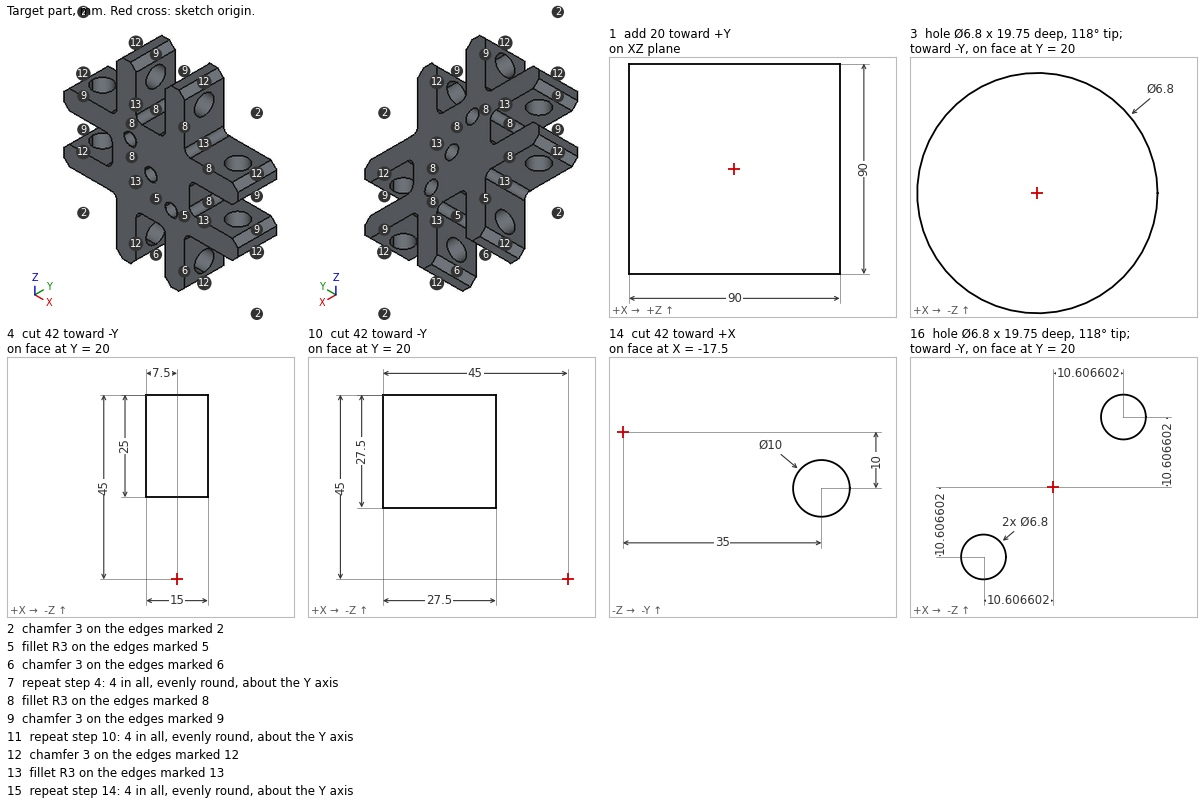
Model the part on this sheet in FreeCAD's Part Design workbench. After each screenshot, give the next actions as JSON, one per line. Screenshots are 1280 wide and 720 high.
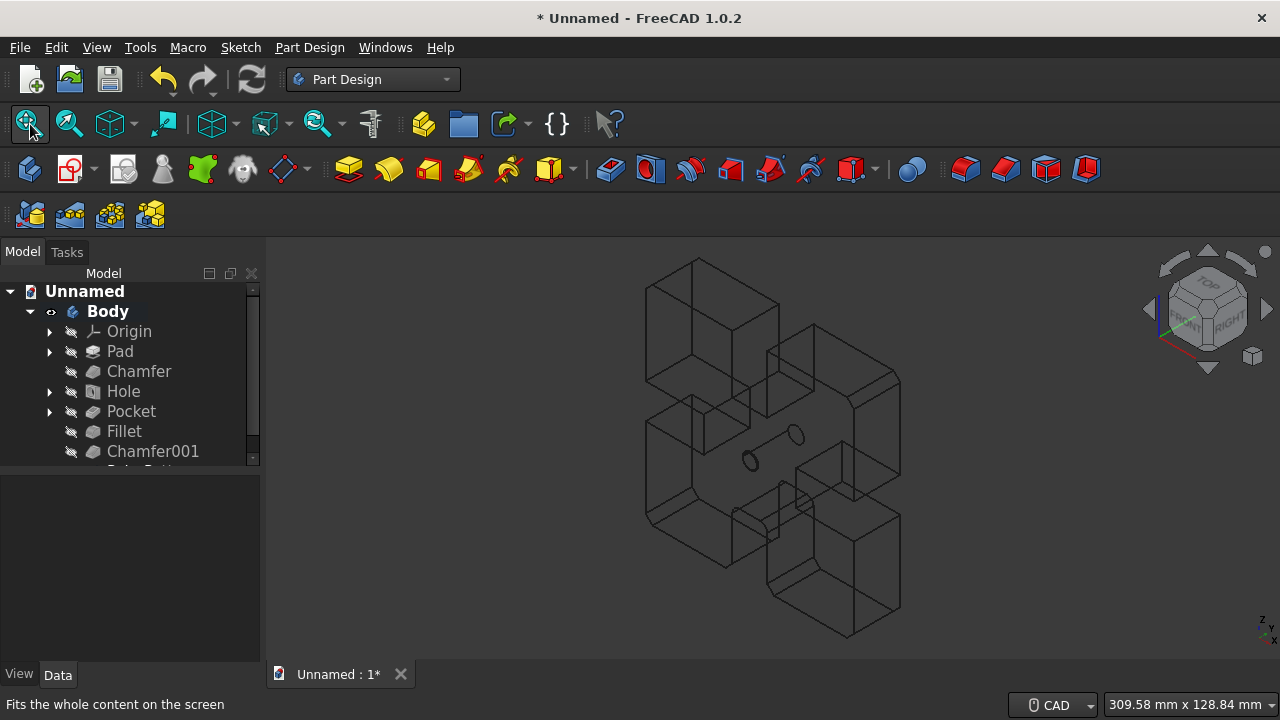
{"action": "left_click", "coordinate": [727, 440]}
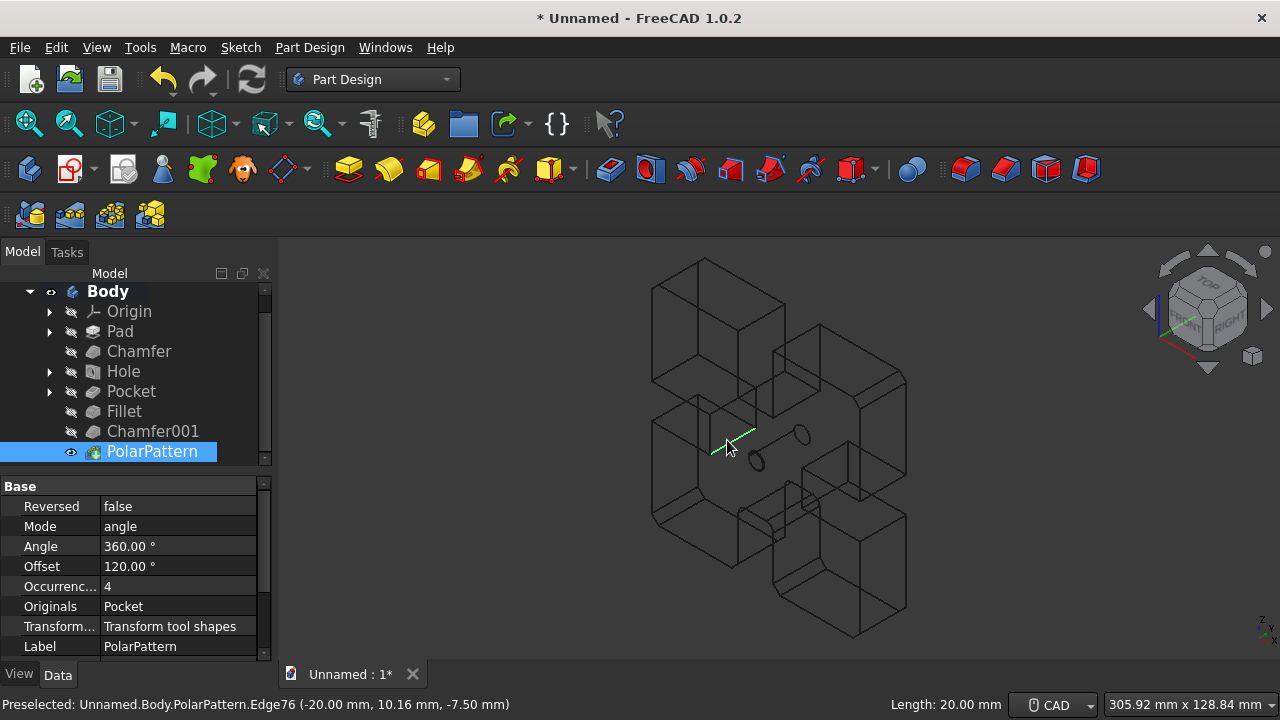
{"action": "left_click", "coordinate": [728, 403], "text": "ctrl"}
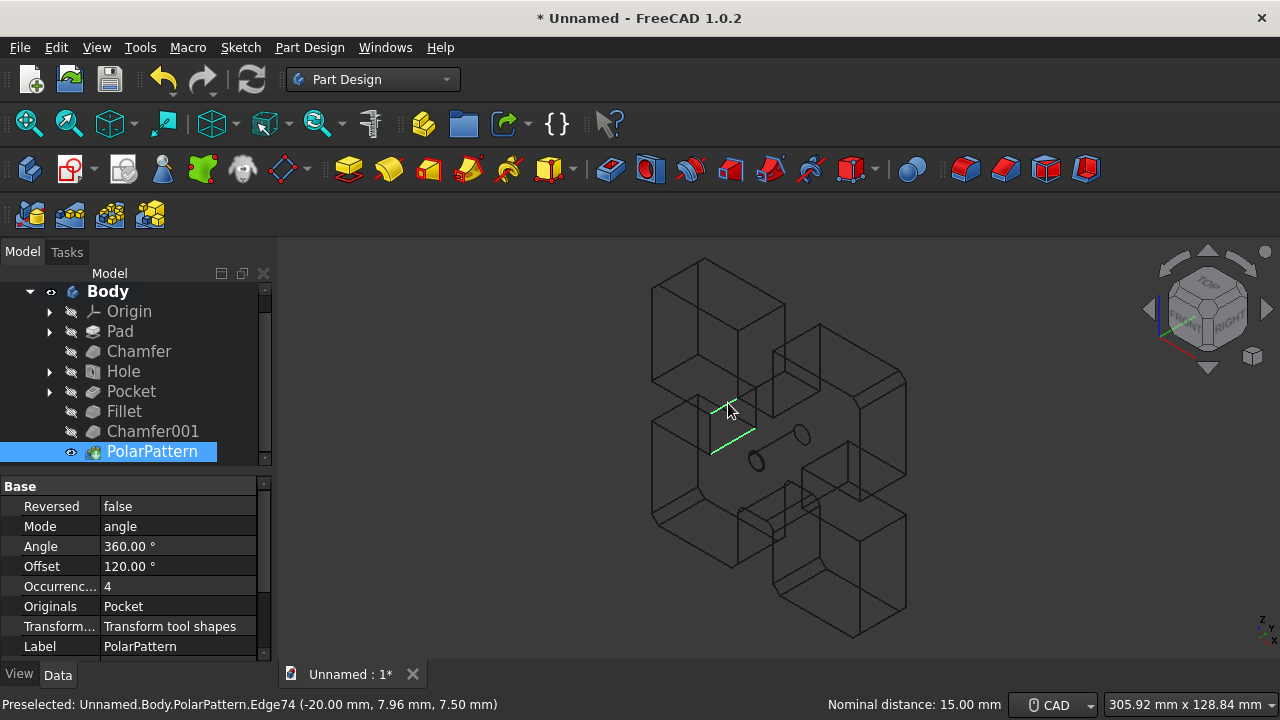
{"action": "left_click", "coordinate": [762, 383], "text": "ctrl"}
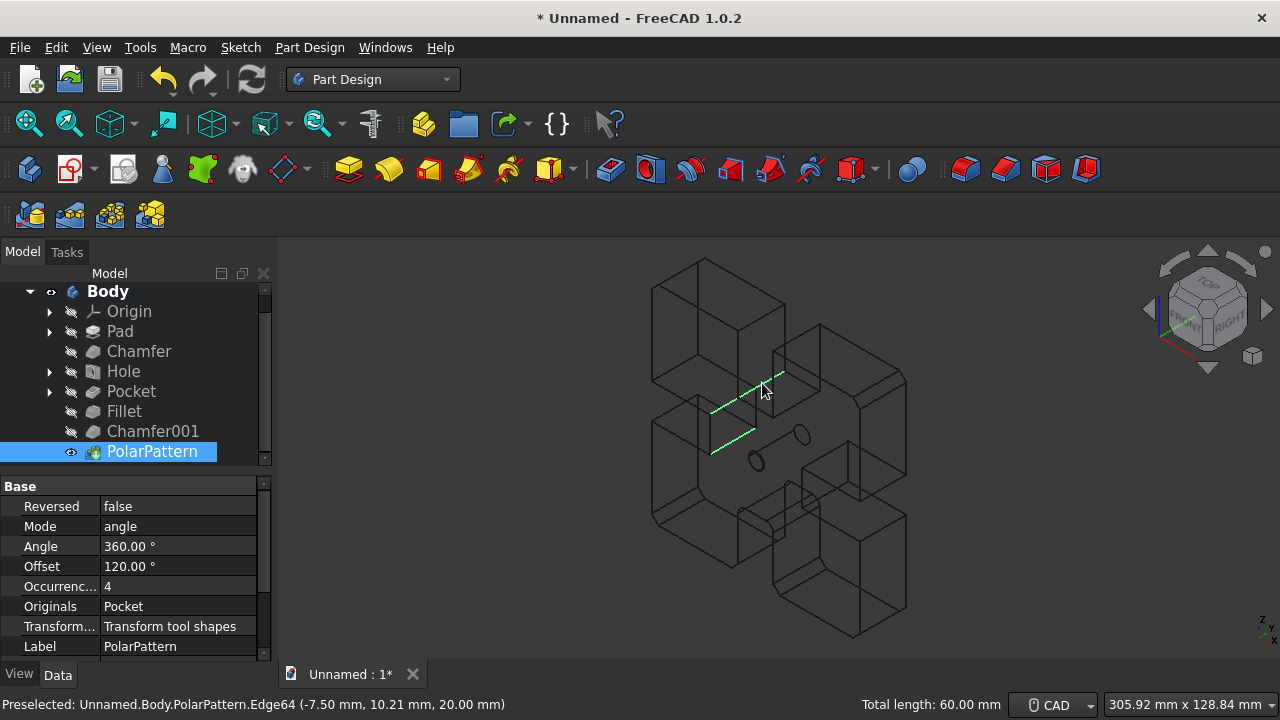
{"action": "left_click", "coordinate": [796, 404], "text": "ctrl"}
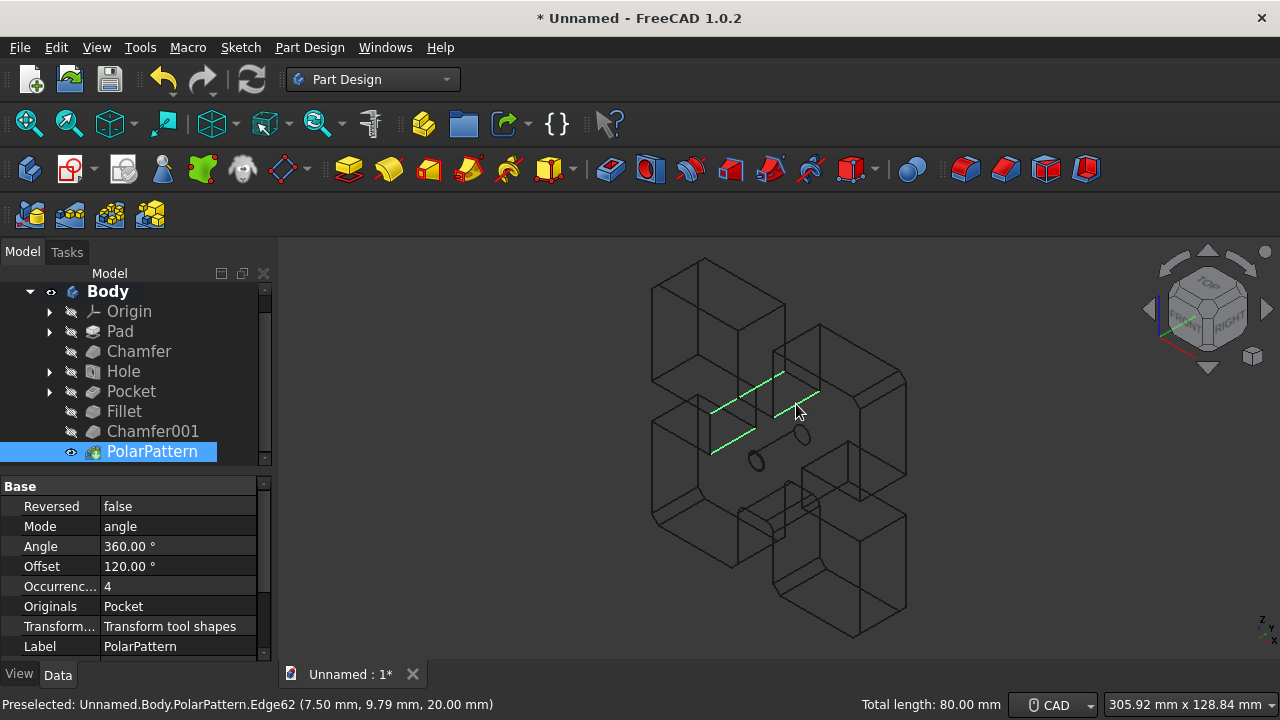
{"action": "left_click", "coordinate": [825, 454], "text": "ctrl"}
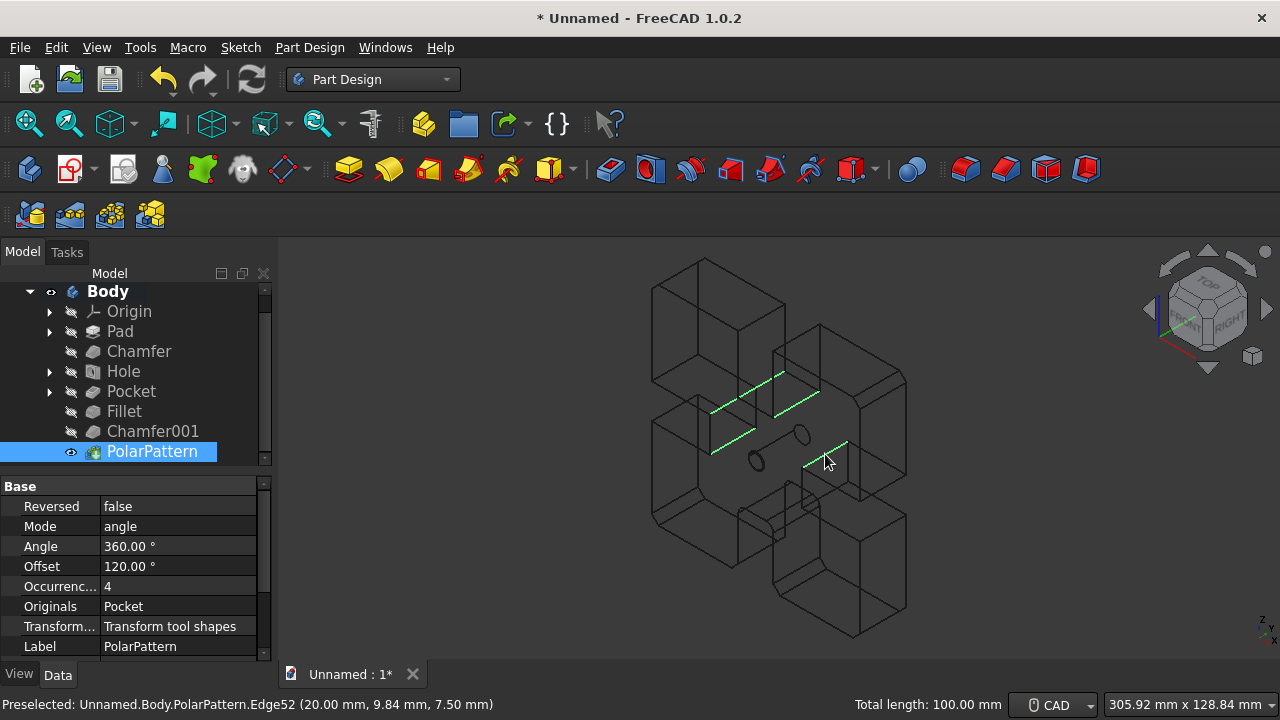
{"action": "left_click", "coordinate": [825, 494], "text": "ctrl"}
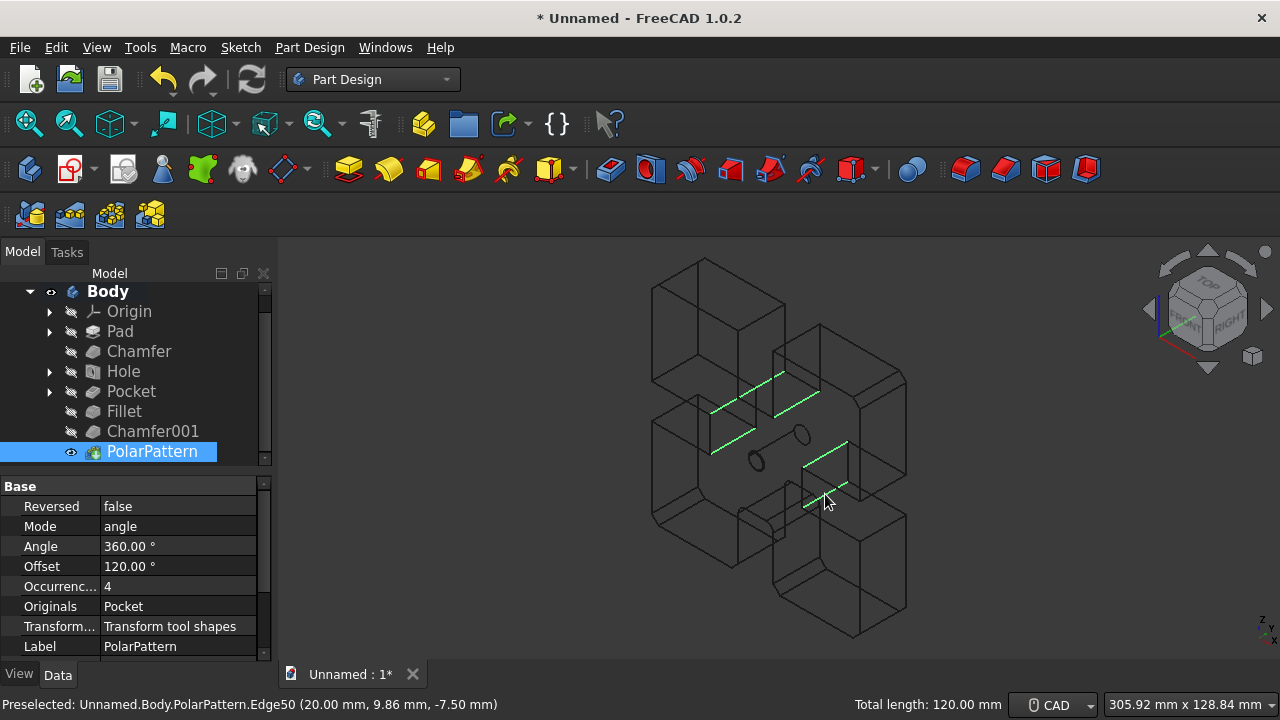
{"action": "key", "text": "v 1"}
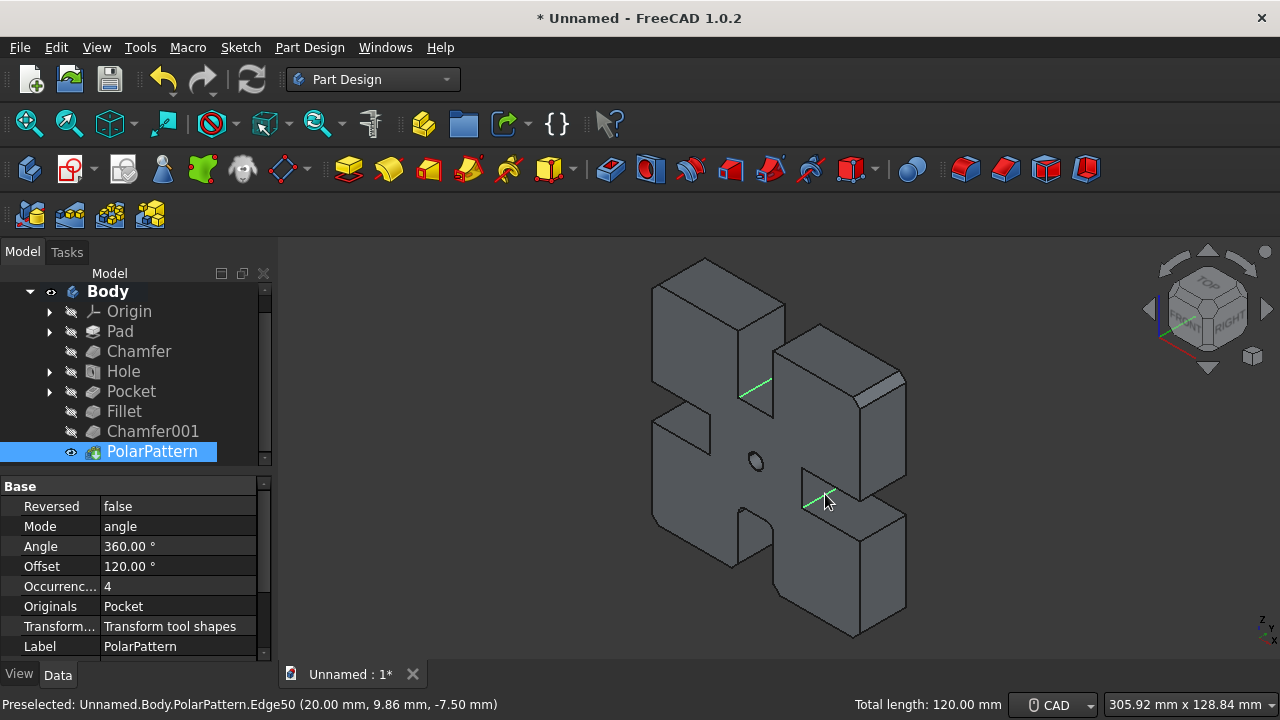
{"action": "left_click", "coordinate": [966, 170]}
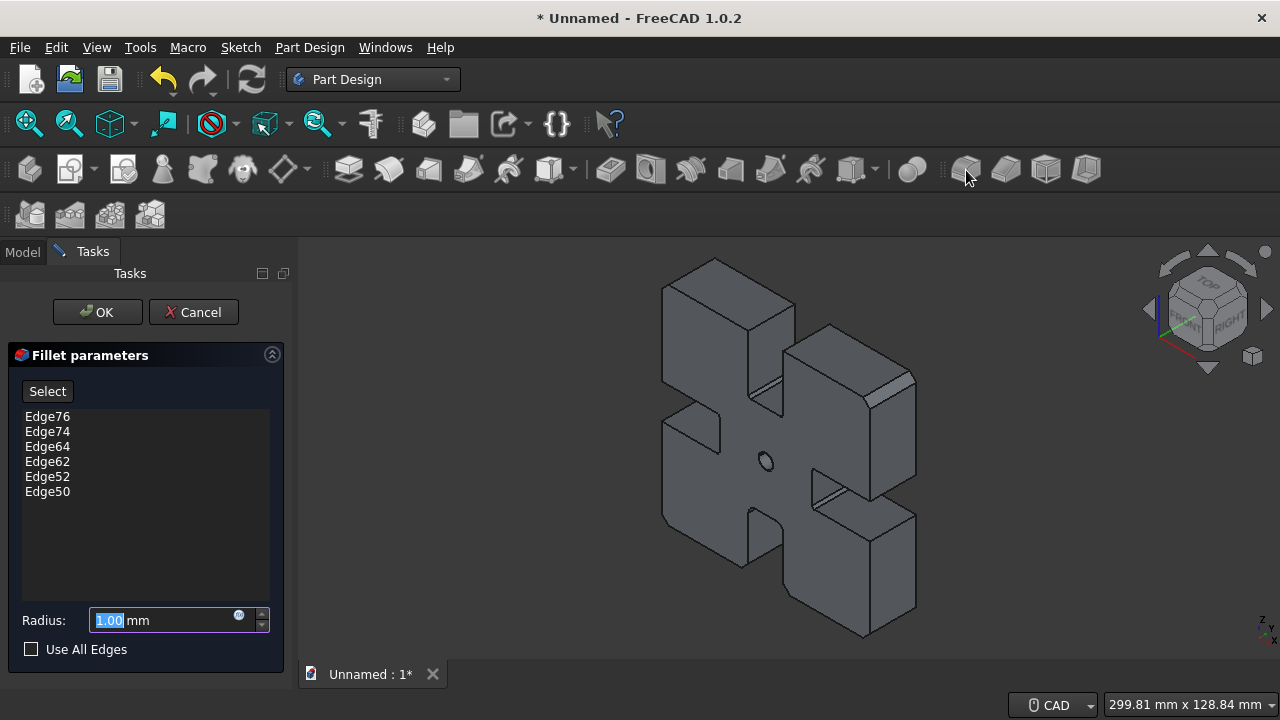
{"action": "type", "text": "3"}
{"action": "key", "text": "Tab"}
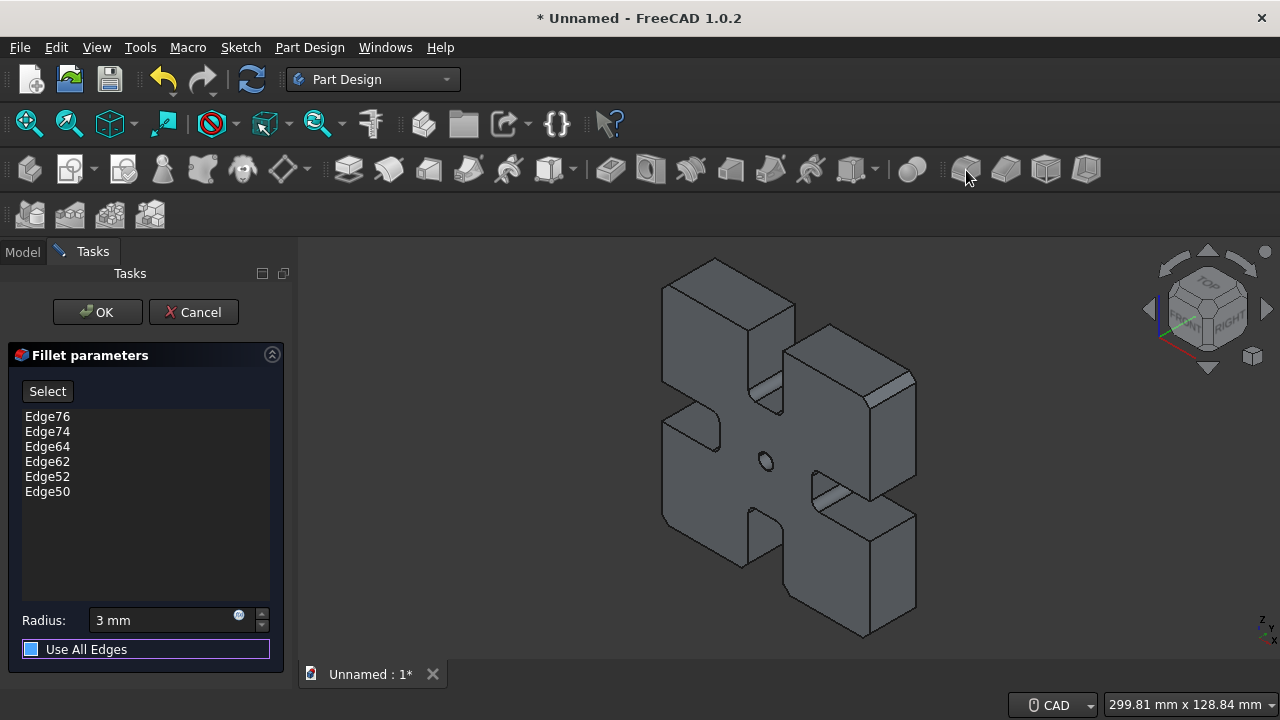
{"action": "left_click", "coordinate": [98, 312]}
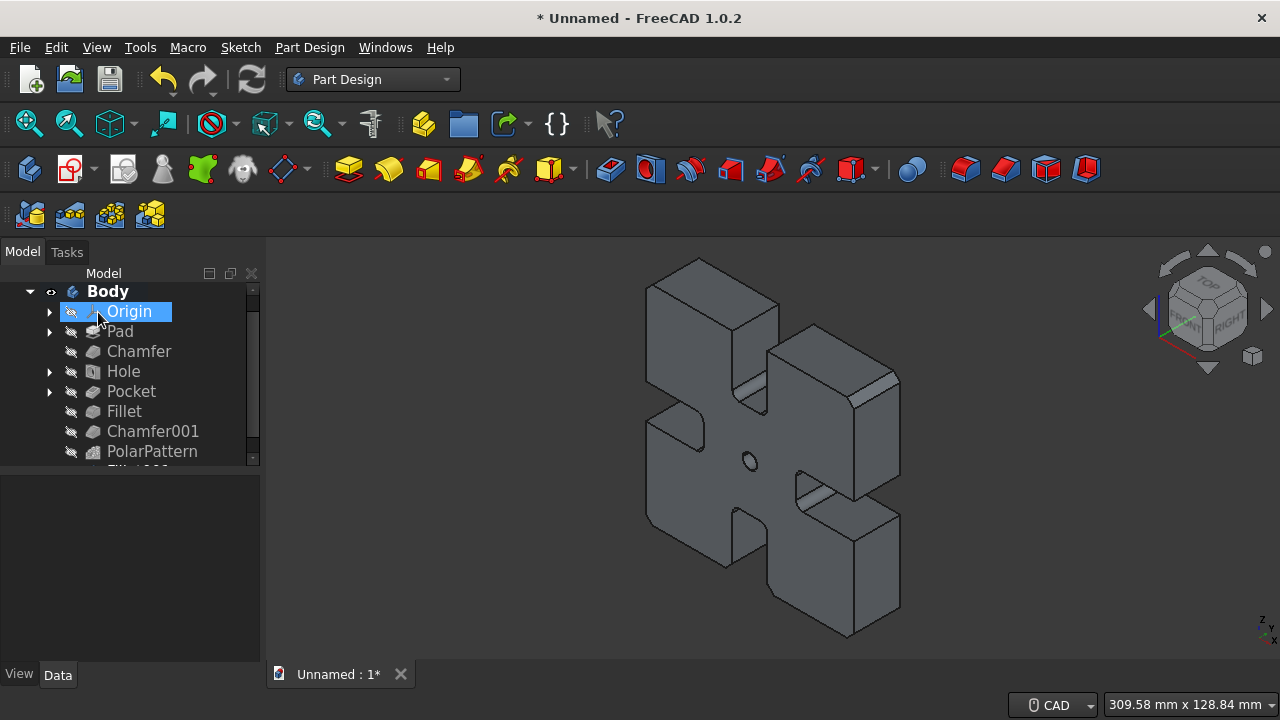
{"action": "left_click", "coordinate": [756, 317]}